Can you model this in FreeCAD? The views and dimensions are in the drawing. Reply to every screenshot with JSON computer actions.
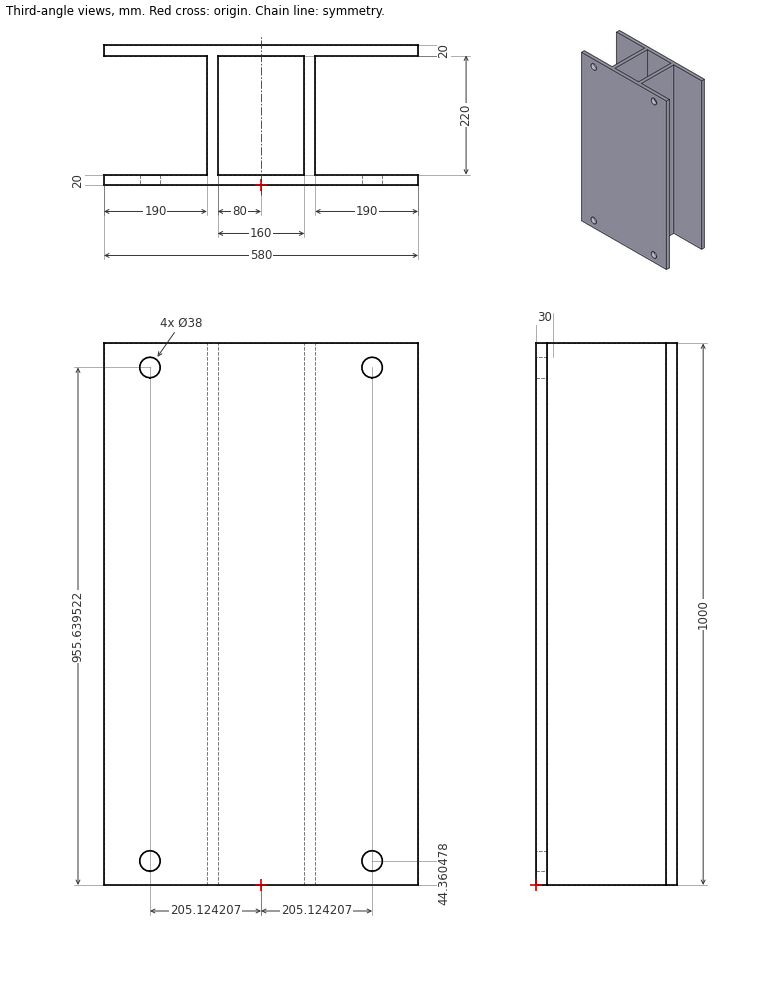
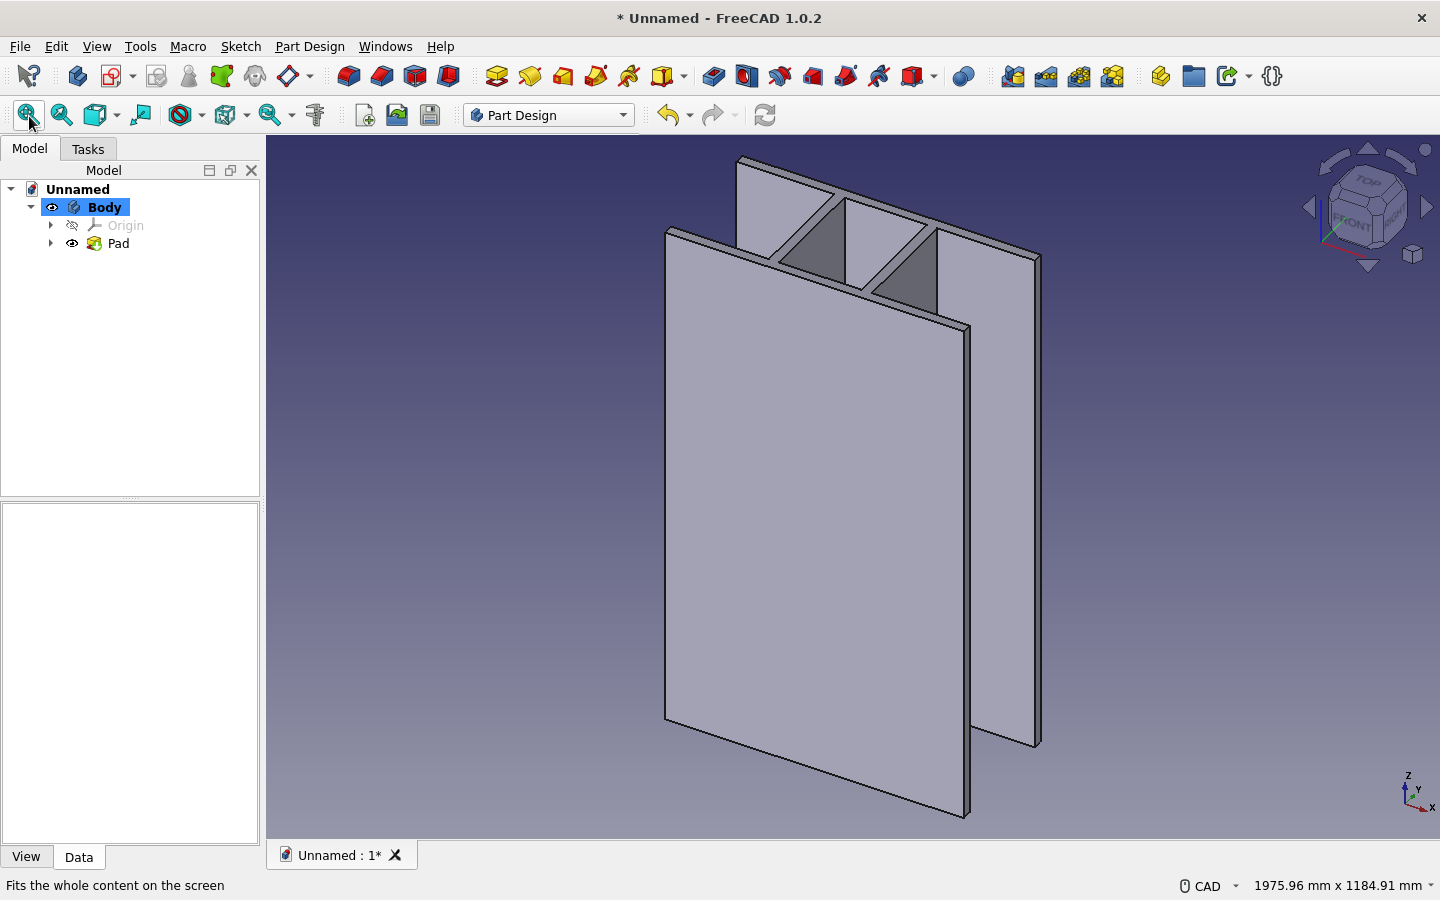
{"action": "left_click", "coordinate": [814, 455]}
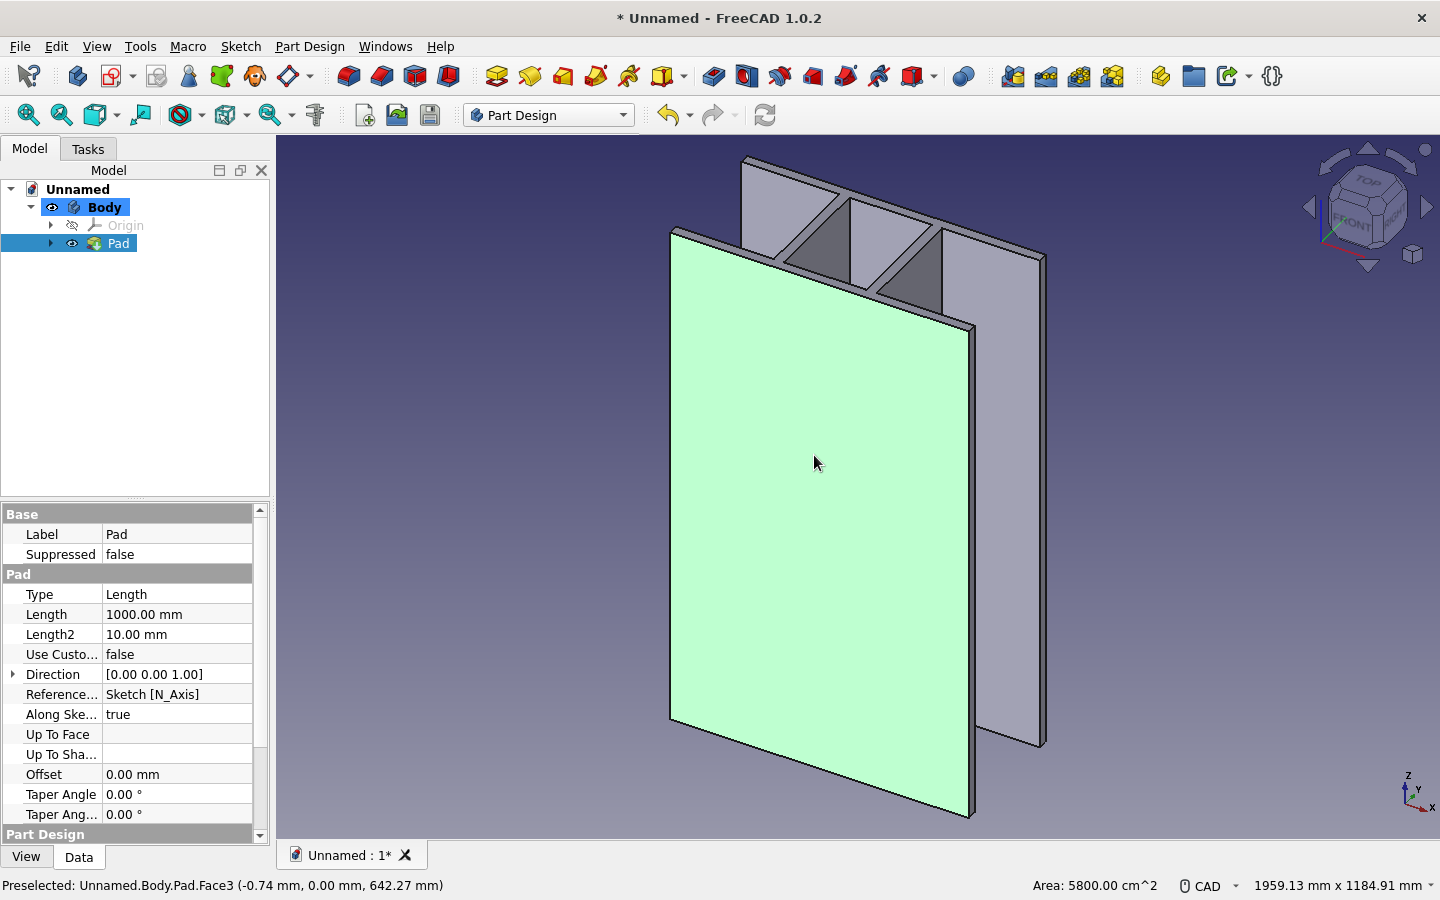
{"action": "left_click", "coordinate": [110, 76]}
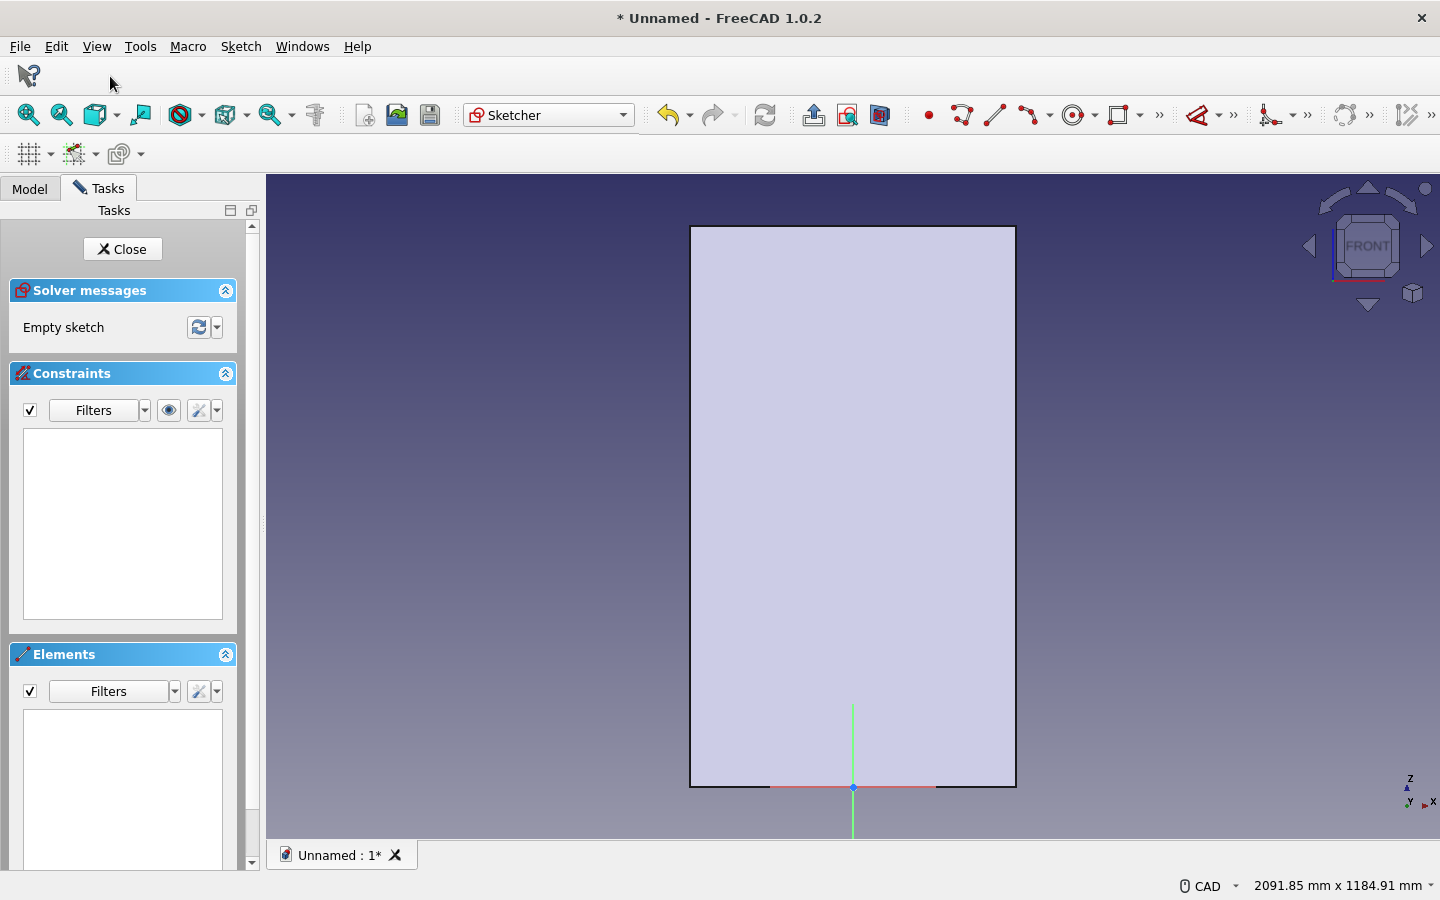
{"action": "scroll", "coordinate": [475, 474], "scroll_direction": "down", "scroll_amount": 1}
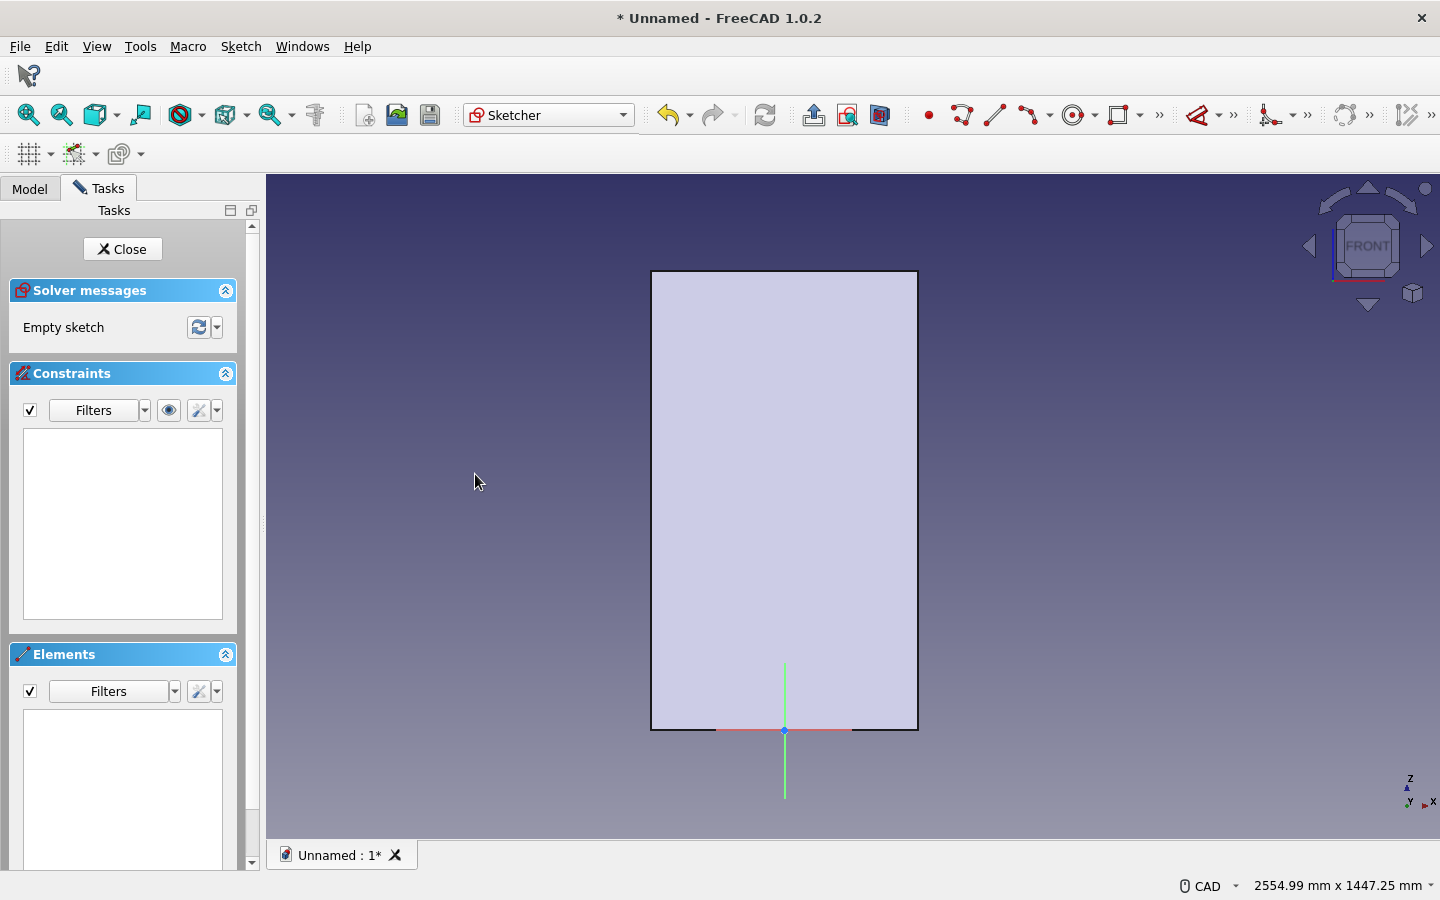
{"action": "key", "text": "g c"}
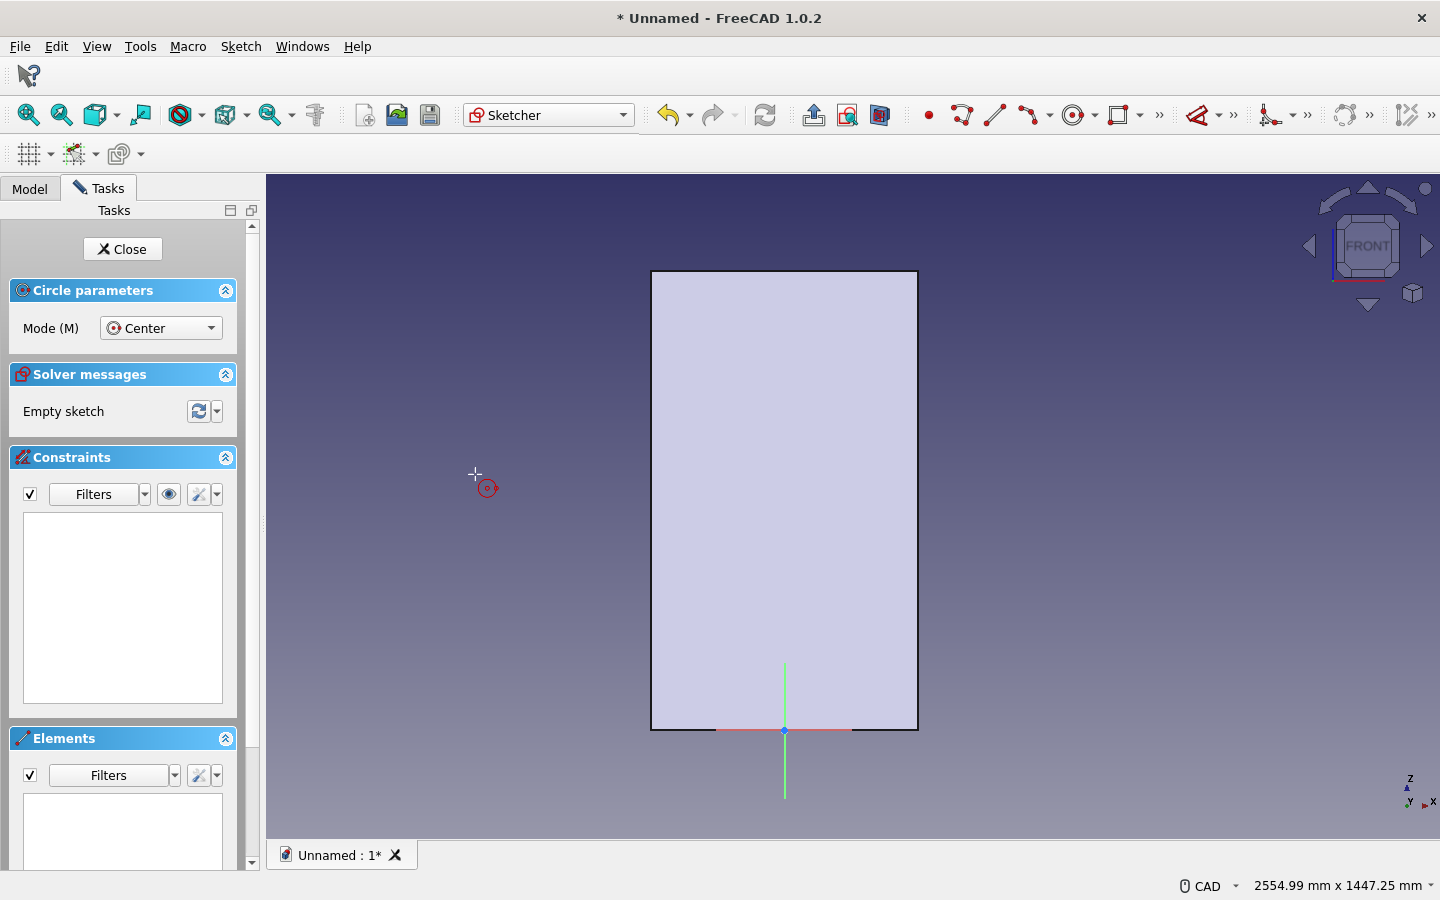
{"action": "scroll", "coordinate": [690, 291], "scroll_direction": "up", "scroll_amount": 5}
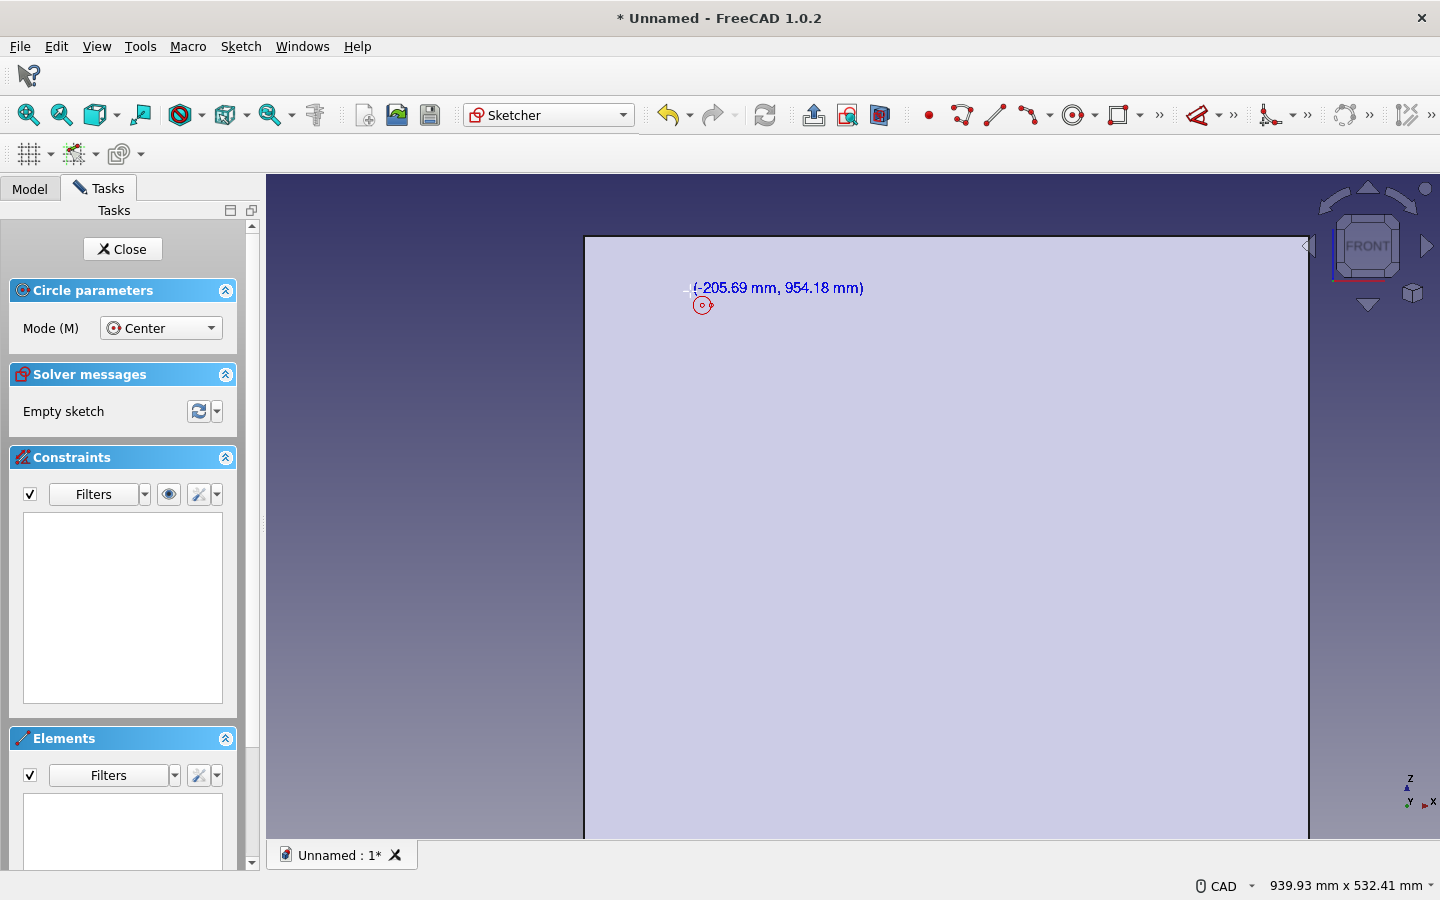
{"action": "left_click", "coordinate": [690, 292]}
{"action": "mouse_move", "coordinate": [707, 275]}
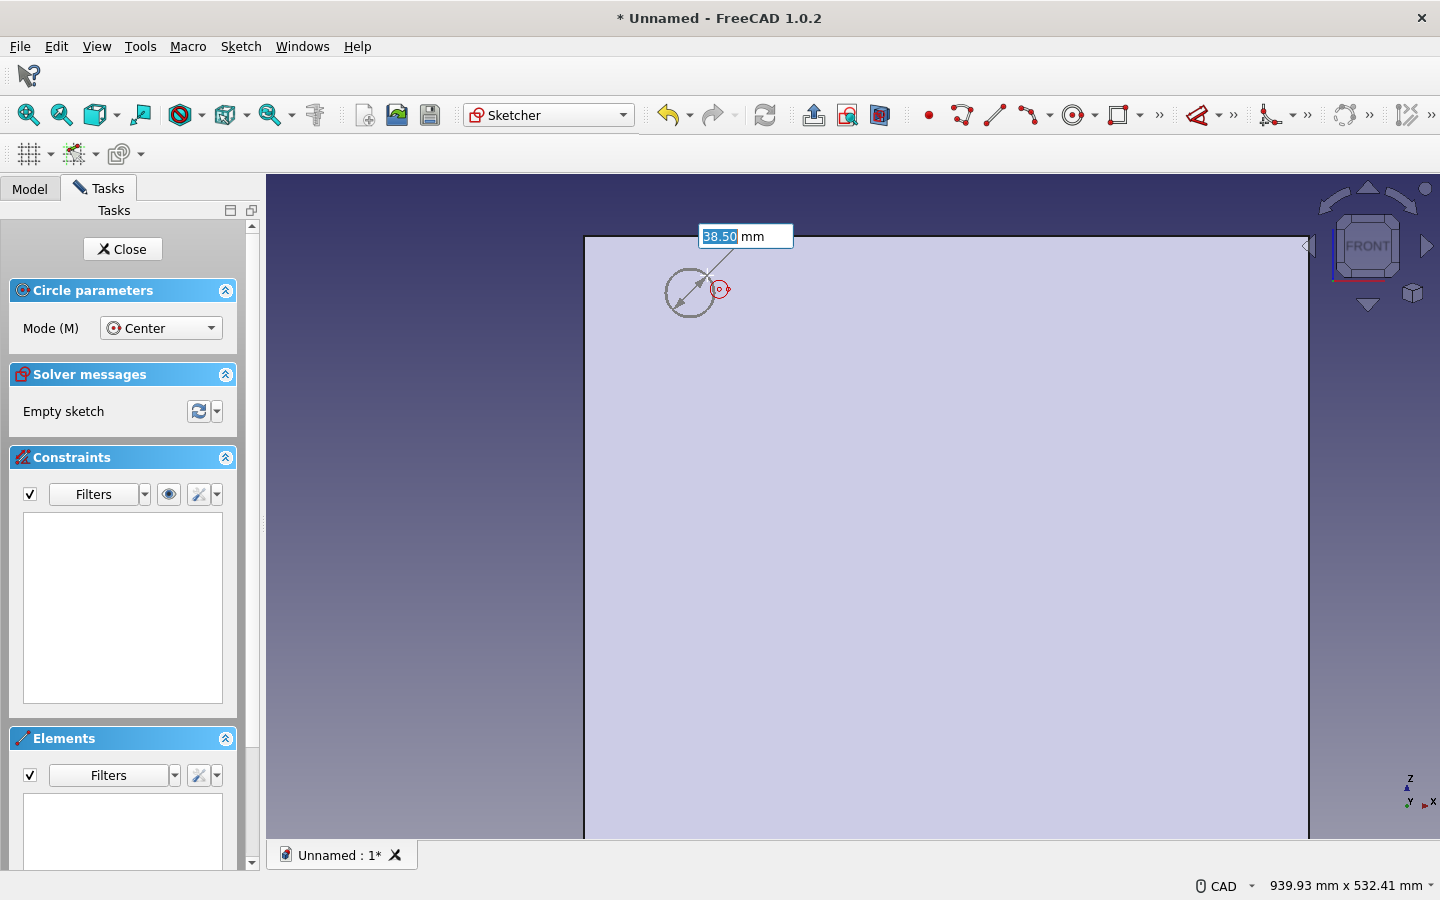
{"action": "type", "text": "38"}
{"action": "key", "text": "Return"}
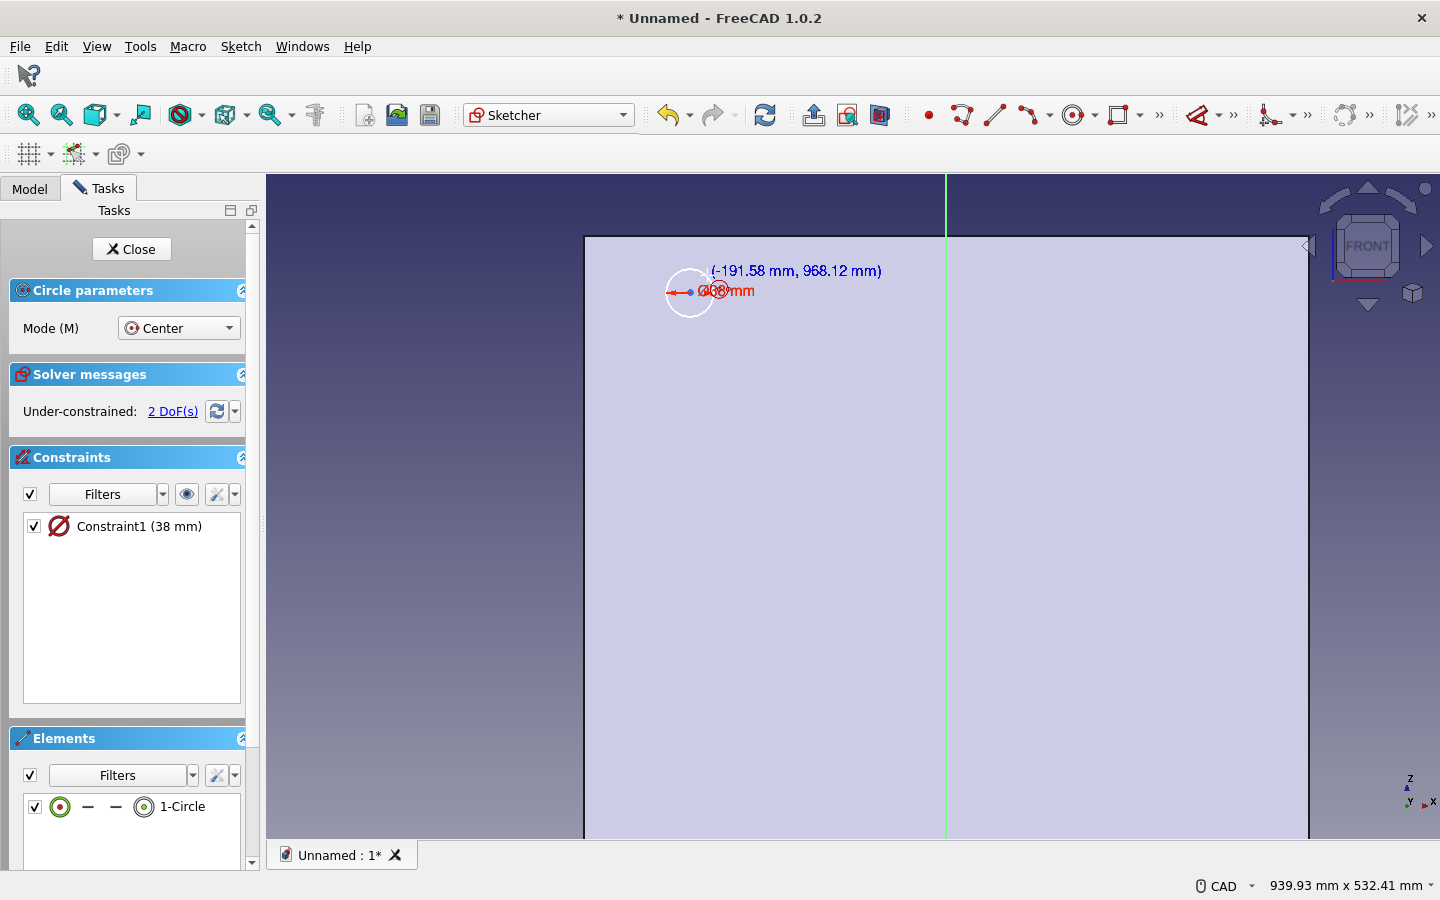
{"action": "left_click", "coordinate": [1202, 292]}
{"action": "mouse_move", "coordinate": [1219, 275]}